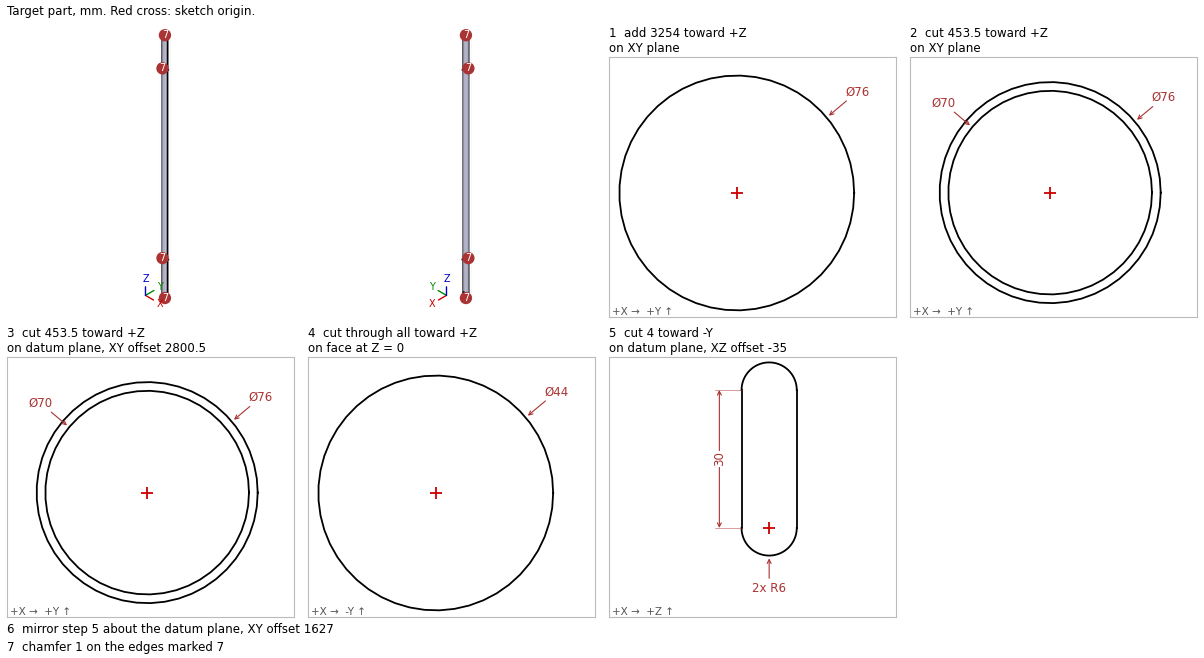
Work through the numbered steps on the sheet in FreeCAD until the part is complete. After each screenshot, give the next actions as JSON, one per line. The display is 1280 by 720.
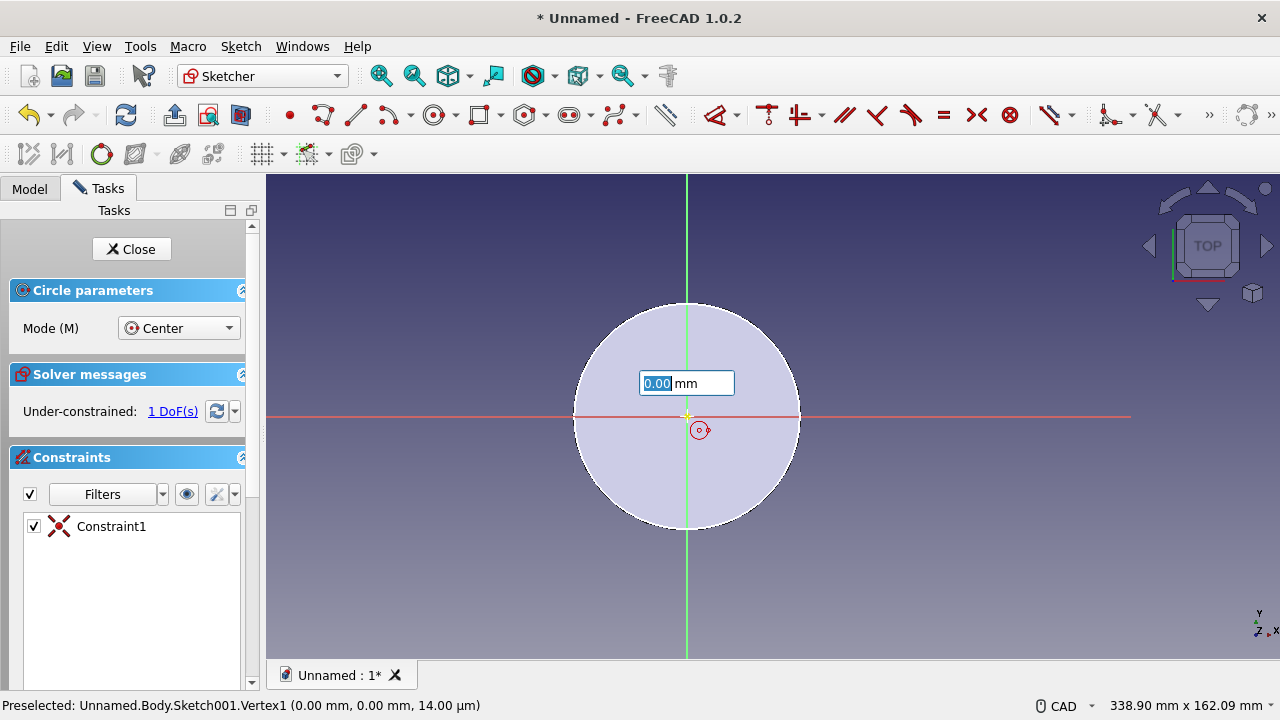
{"action": "scroll", "coordinate": [761, 342], "scroll_direction": "up", "scroll_amount": 3}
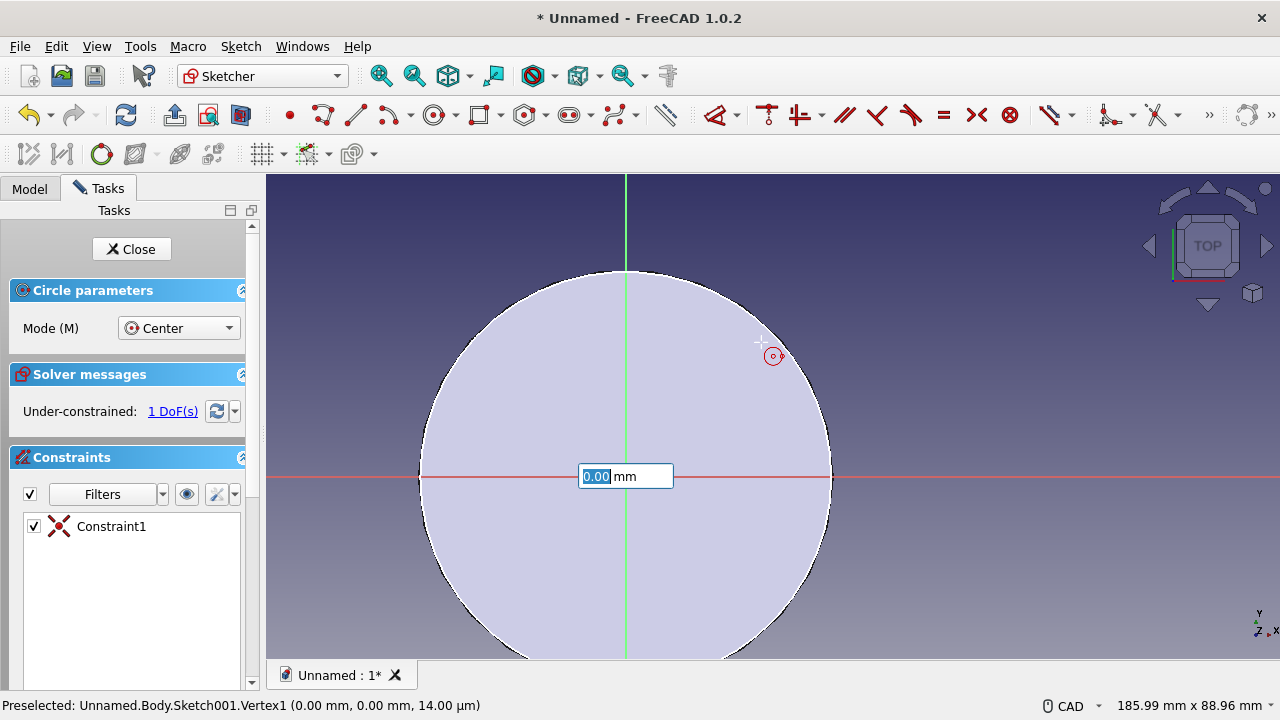
{"action": "left_click", "coordinate": [761, 343]}
{"action": "key", "text": "Escape"}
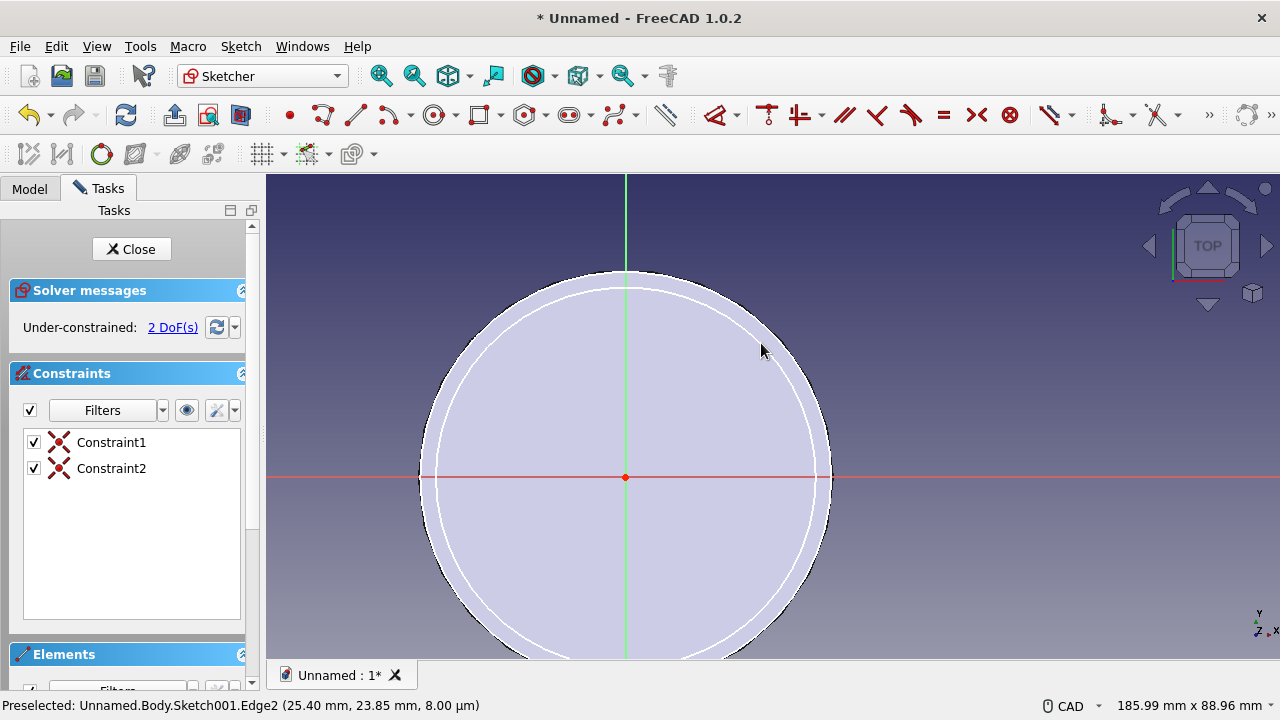
{"action": "left_click", "coordinate": [771, 332]}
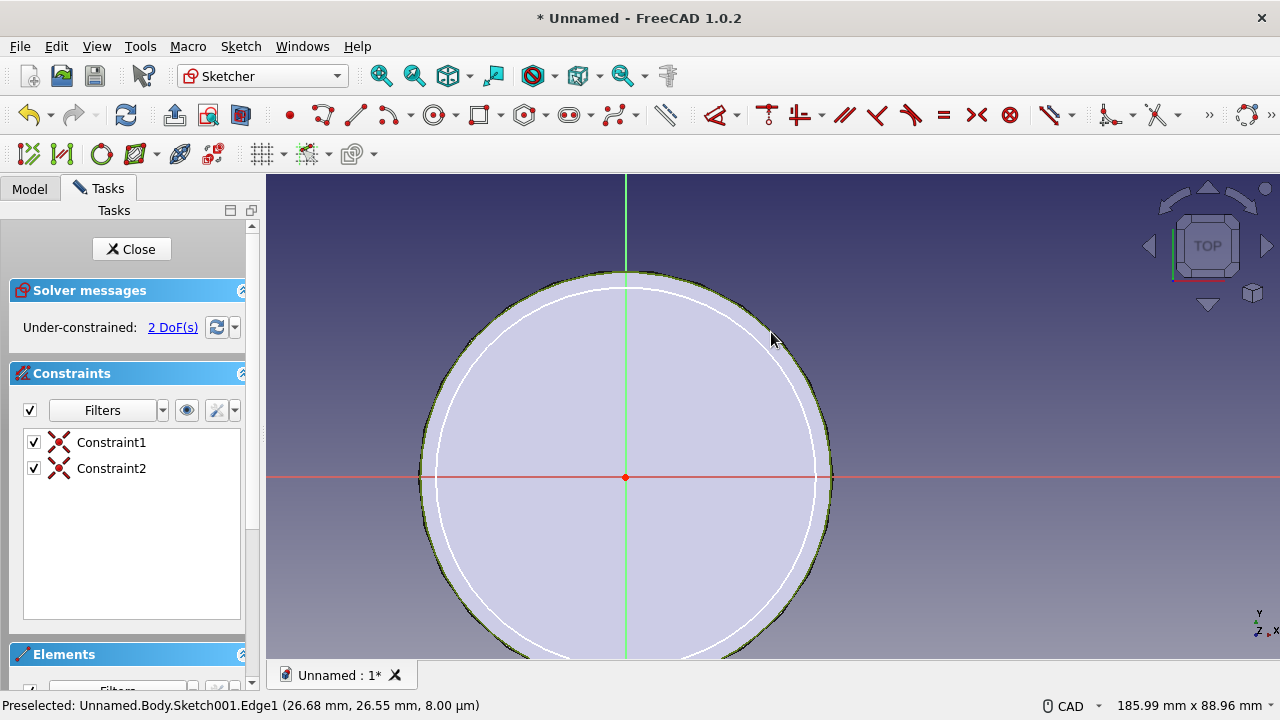
{"action": "left_click", "coordinate": [736, 116]}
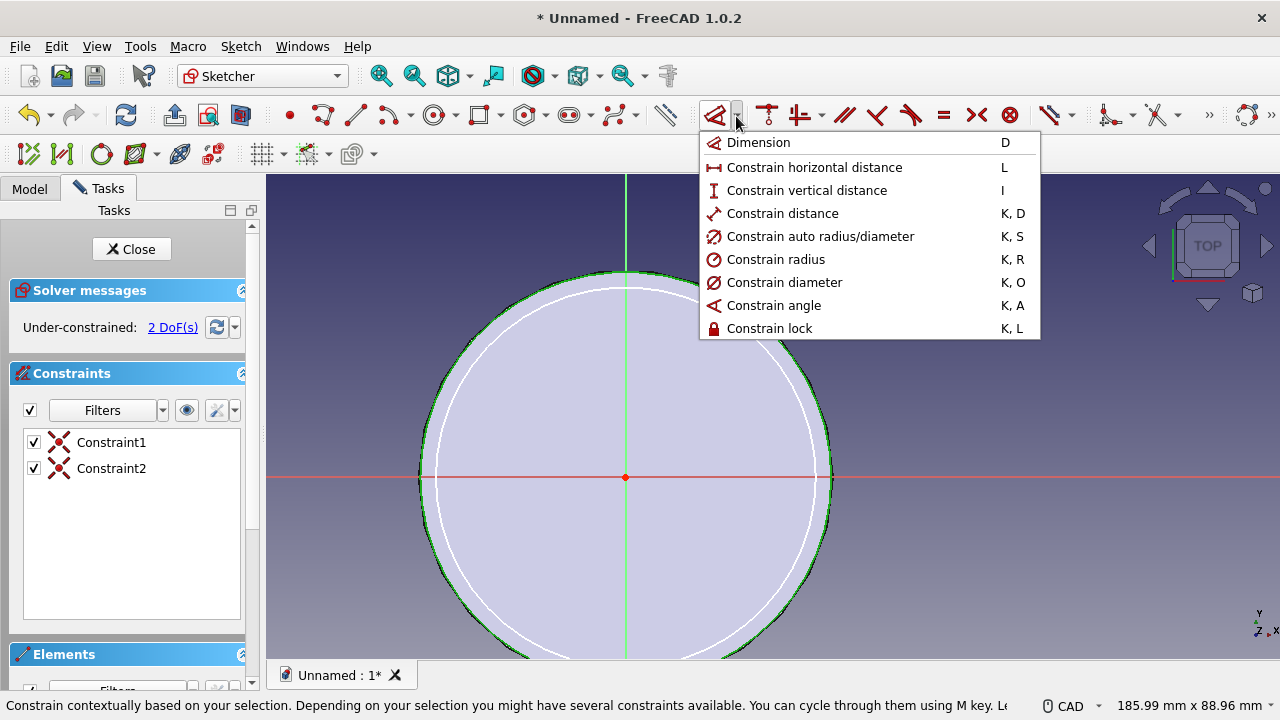
{"action": "left_click", "coordinate": [870, 282]}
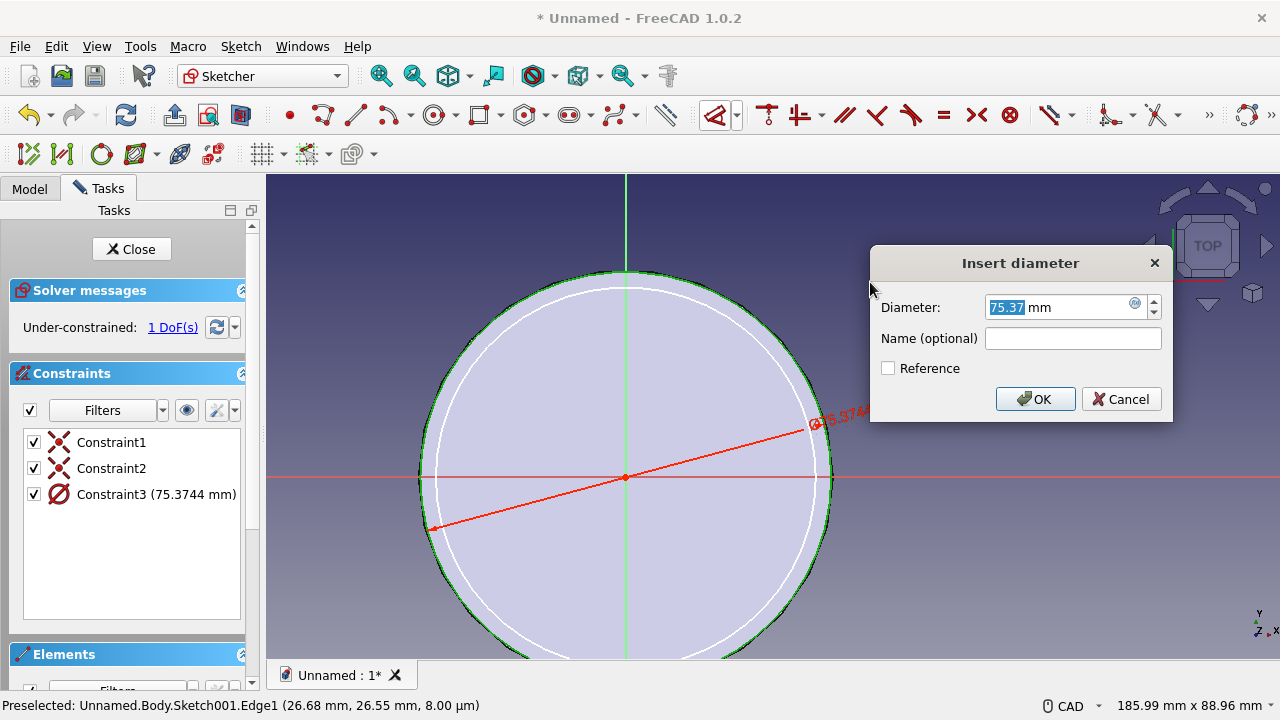
{"action": "type", "text": "76"}
{"action": "key", "text": "Return"}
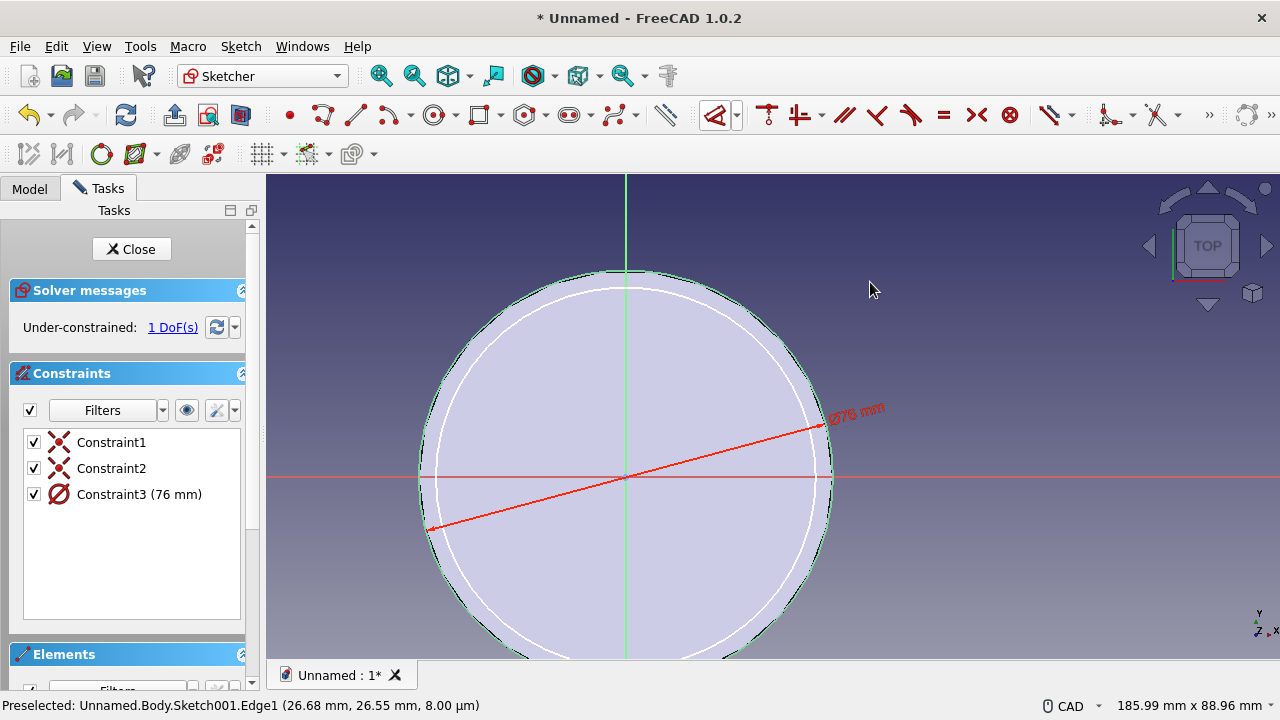
{"action": "left_click", "coordinate": [760, 343]}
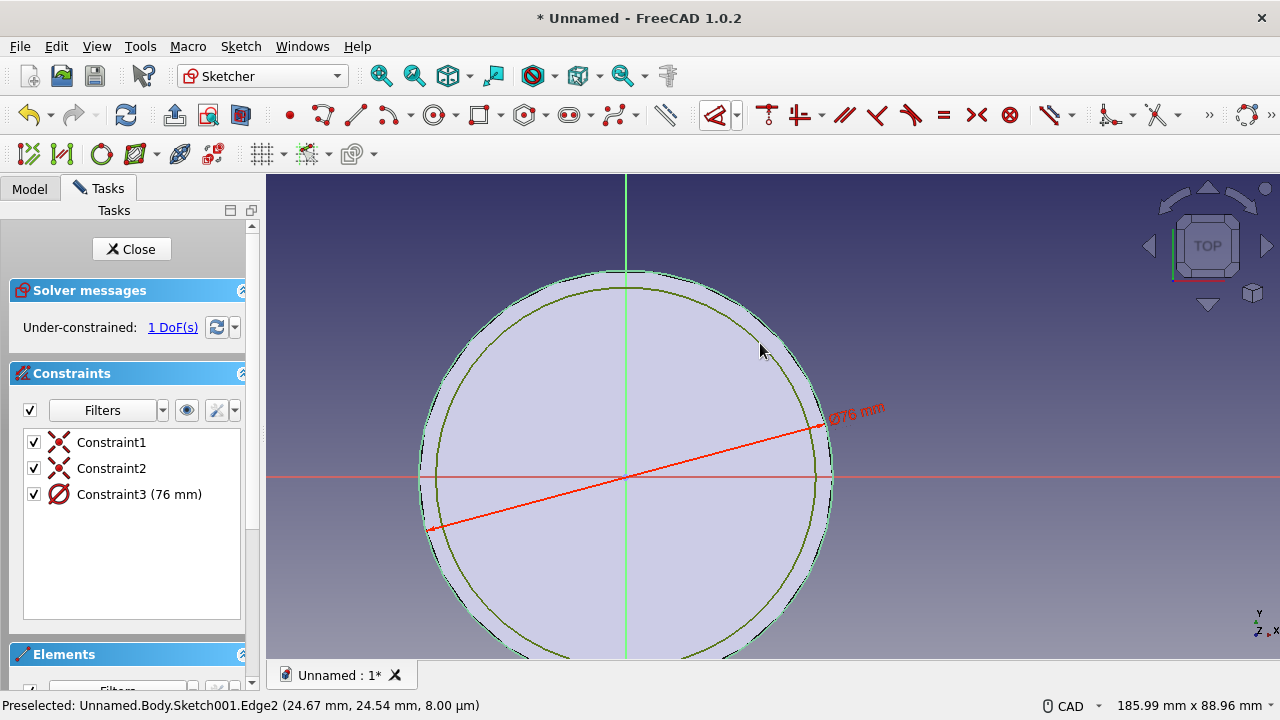
{"action": "left_click", "coordinate": [736, 116]}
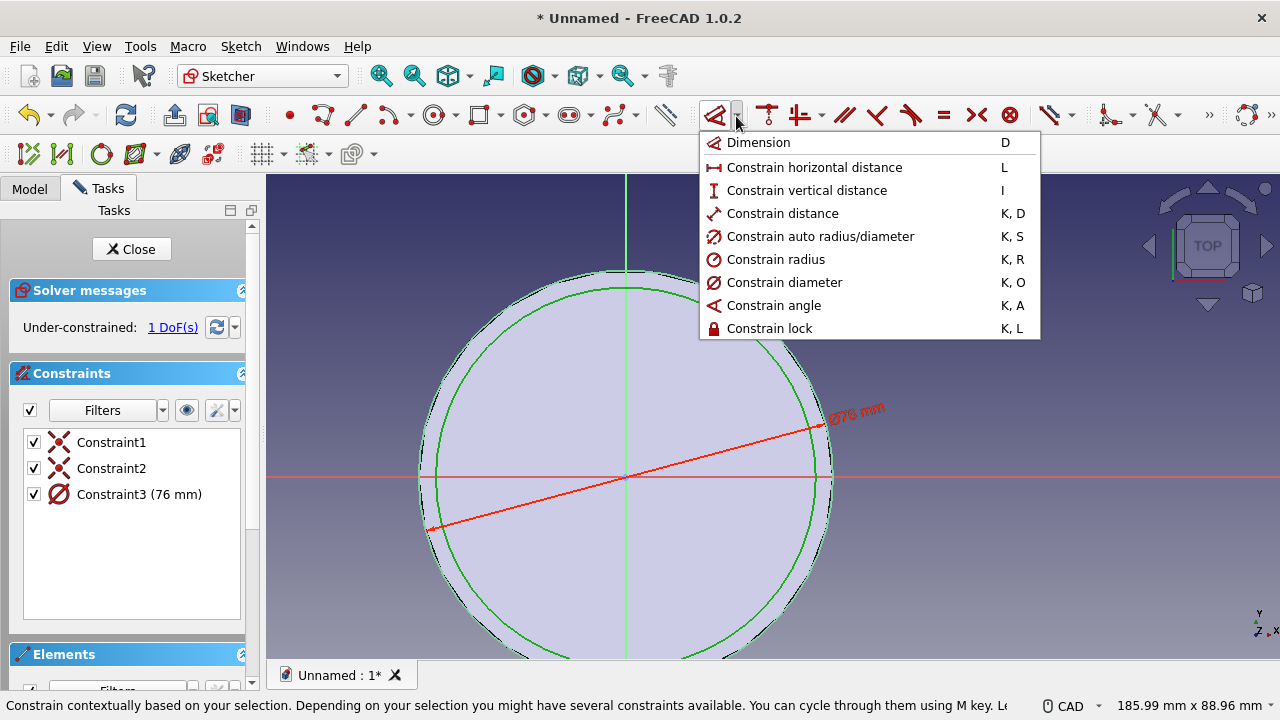
{"action": "left_click", "coordinate": [870, 282]}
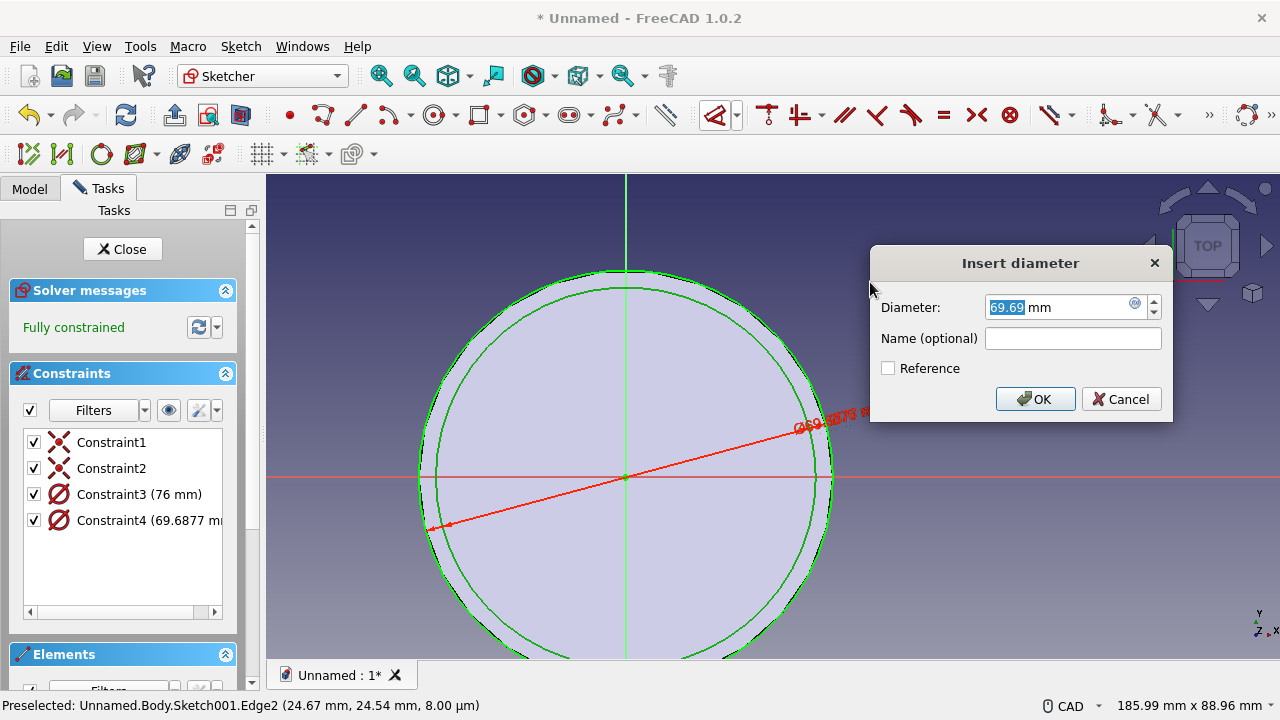
{"action": "type", "text": "70"}
{"action": "key", "text": "Return"}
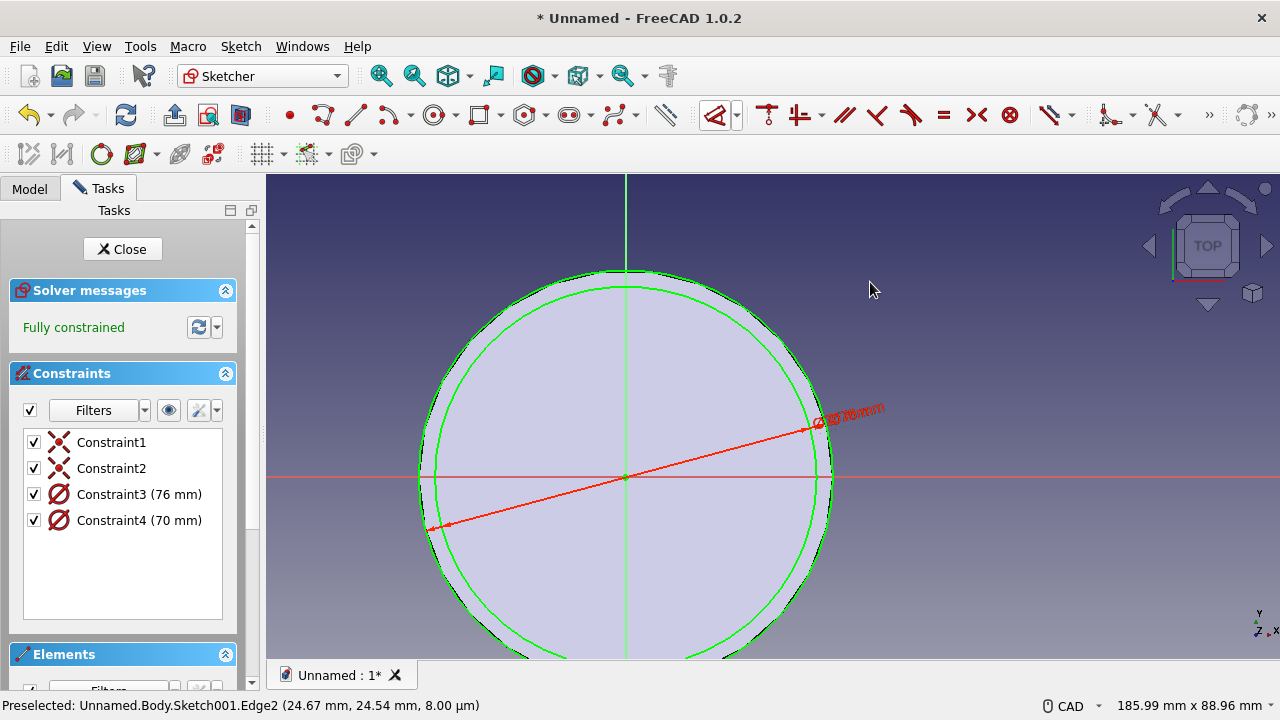
{"action": "left_click", "coordinate": [123, 249]}